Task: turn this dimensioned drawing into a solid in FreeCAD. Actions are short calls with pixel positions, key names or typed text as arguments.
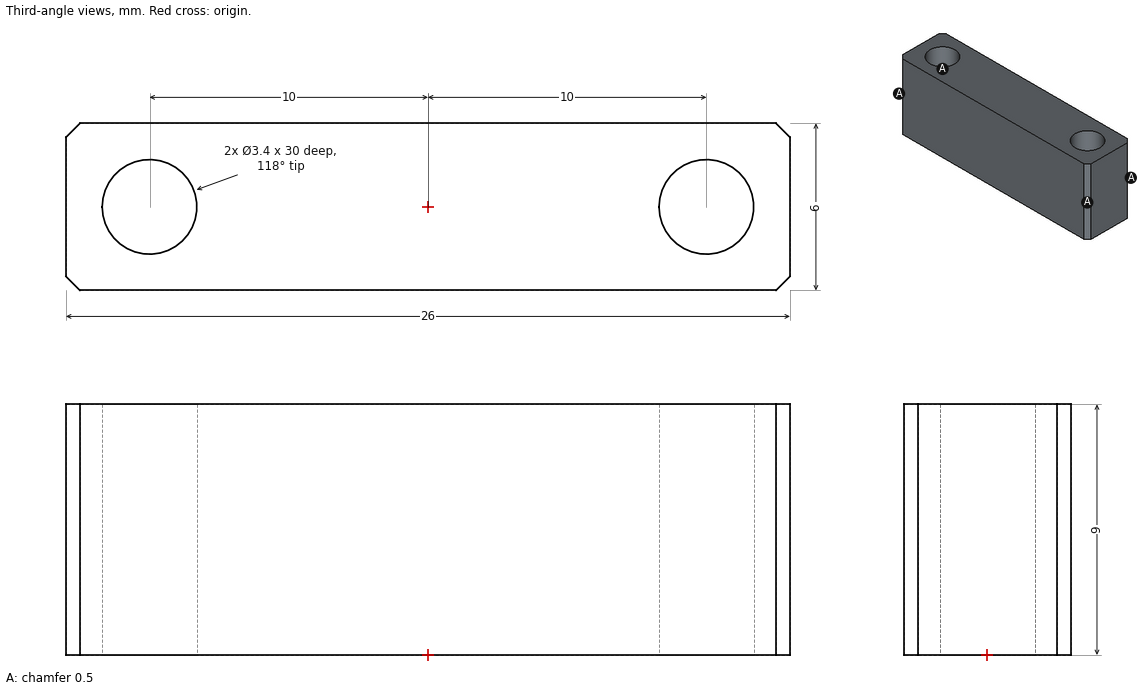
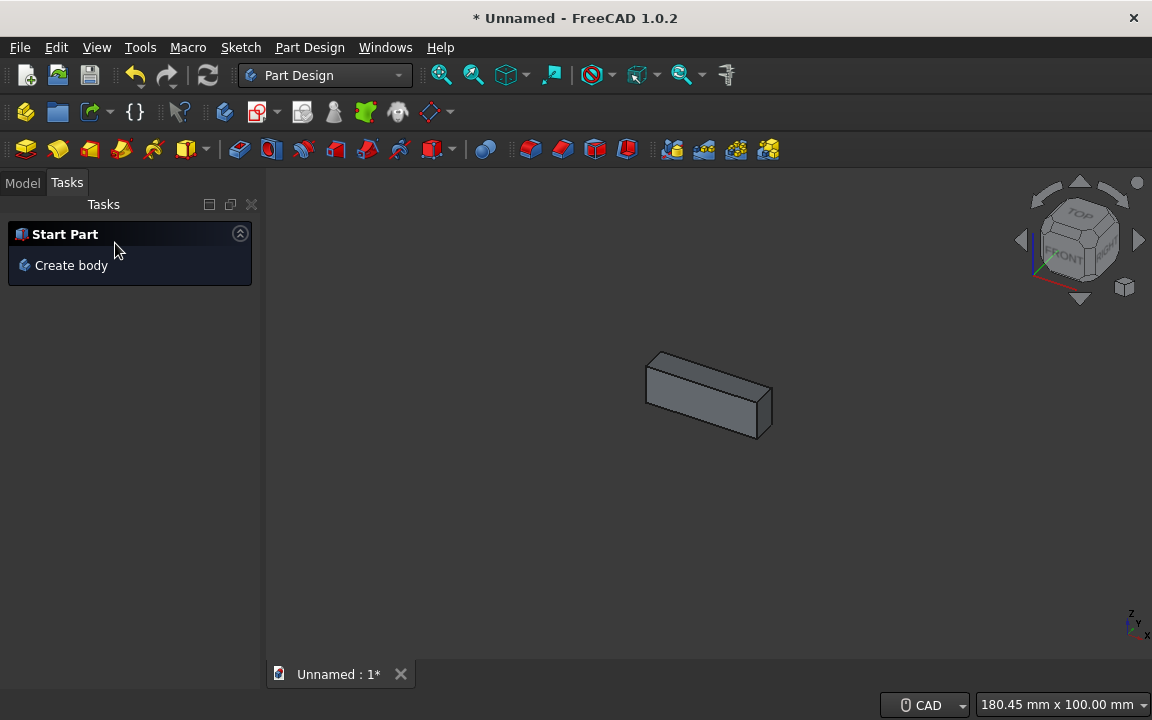
key(v)
key(f)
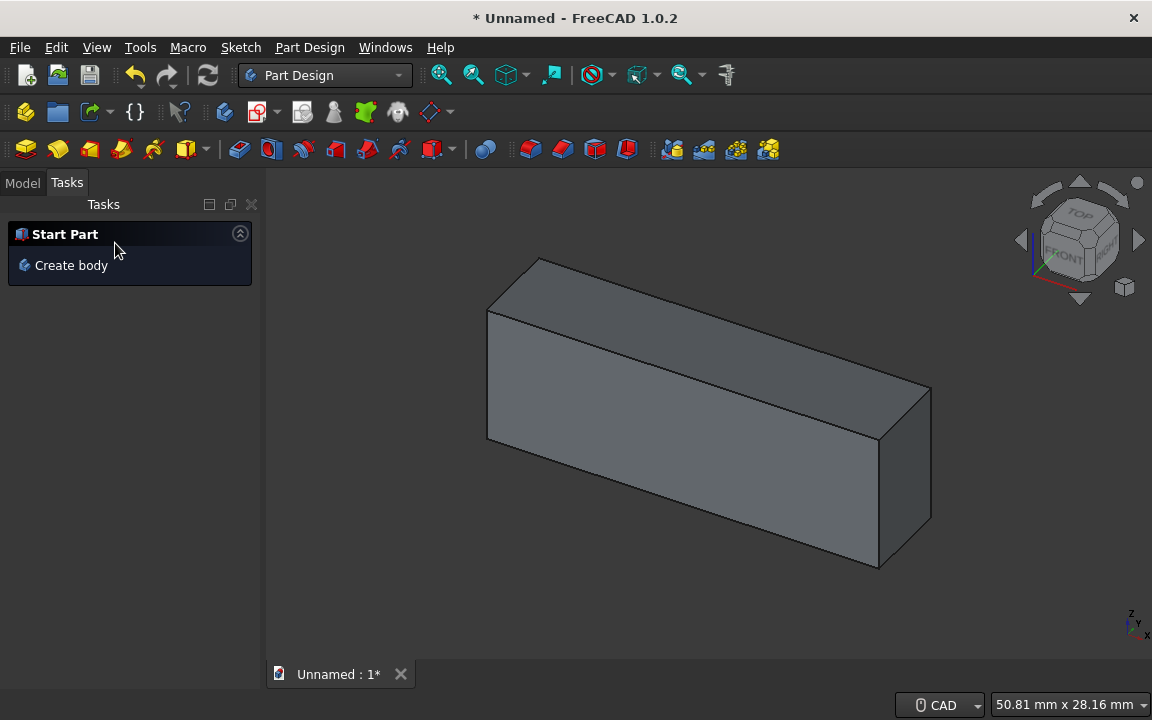
click(821, 385)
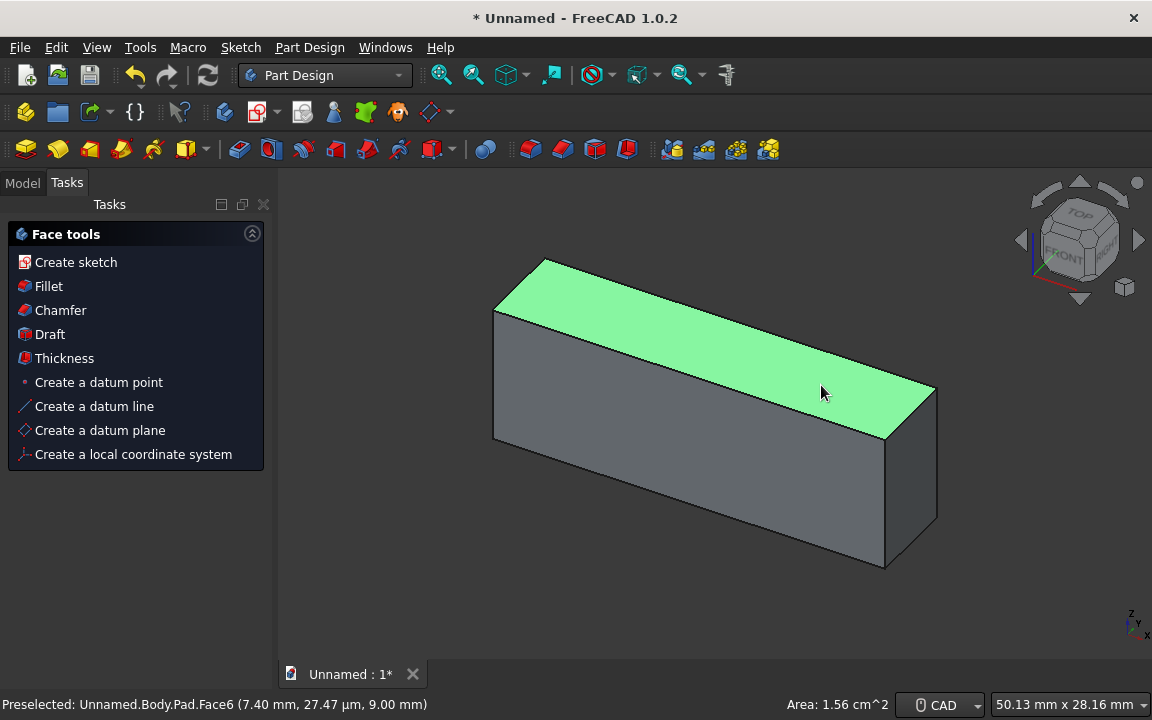
click(258, 112)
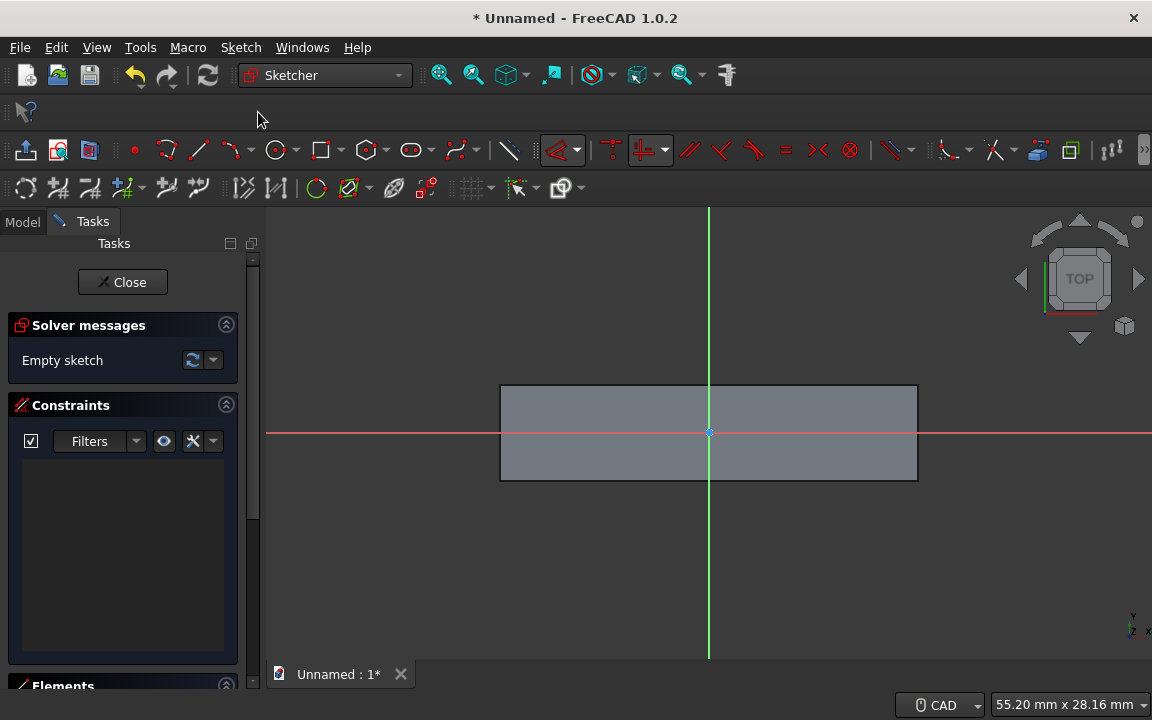
click(276, 150)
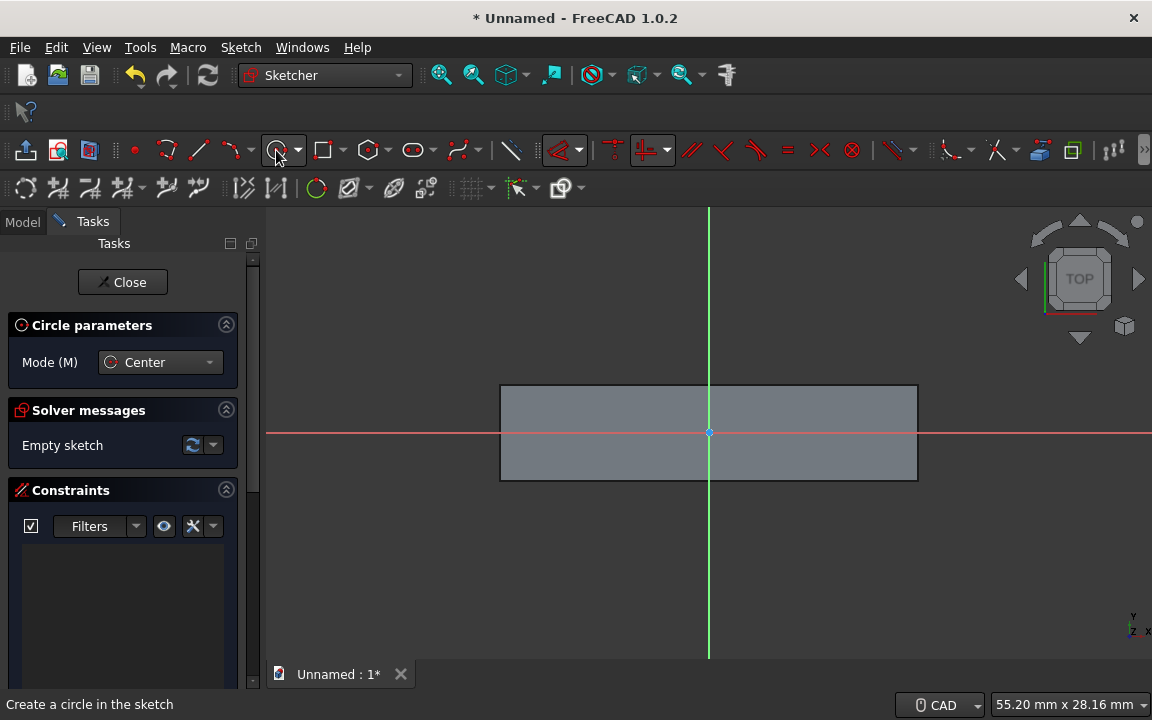
click(548, 433)
move(568, 414)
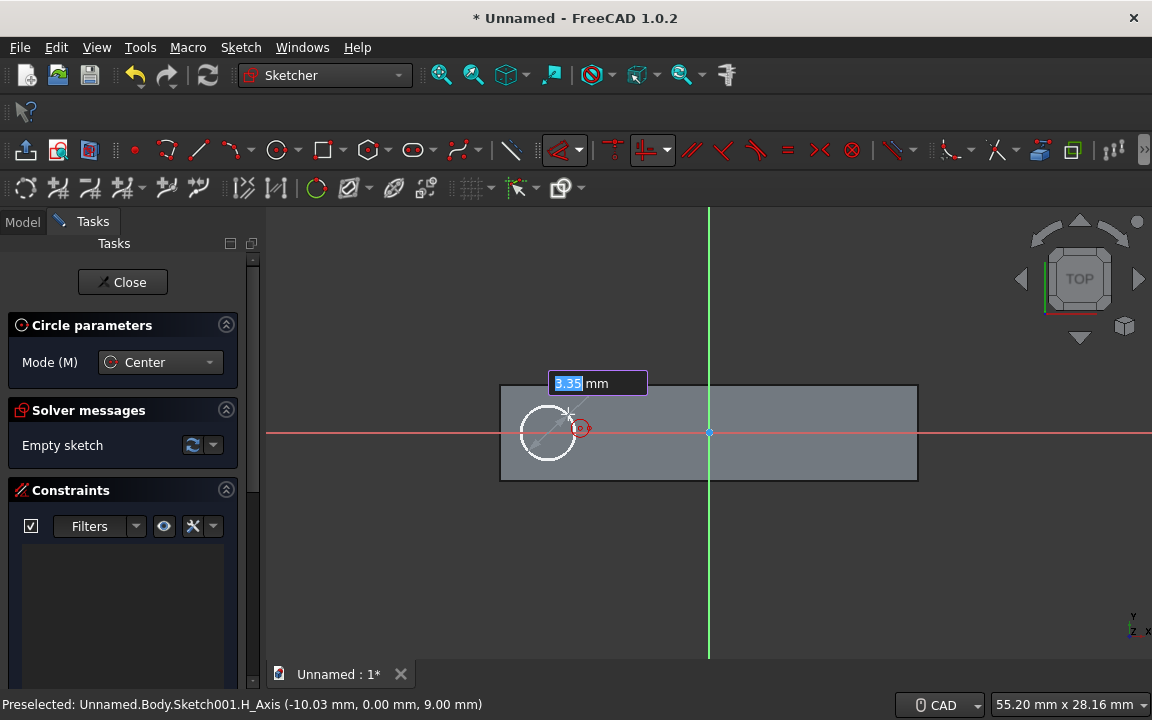
text(3.4)
key(Return)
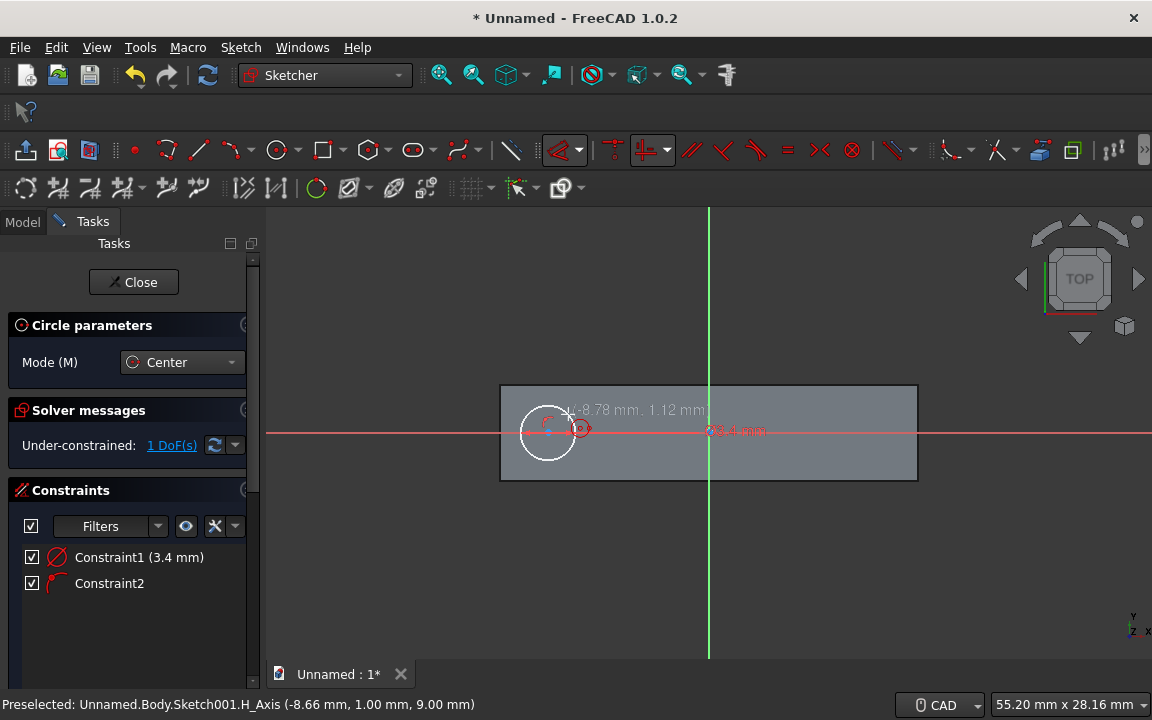
click(870, 433)
move(889, 414)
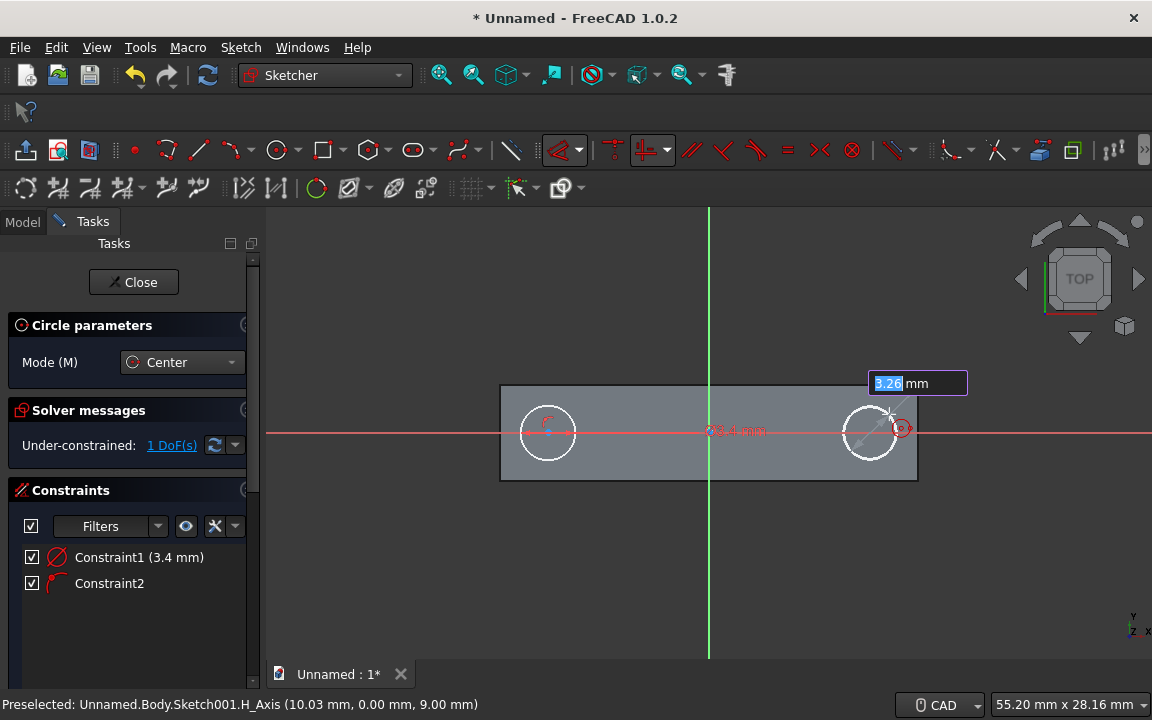
text(3.4)
key(Return)
key(Escape)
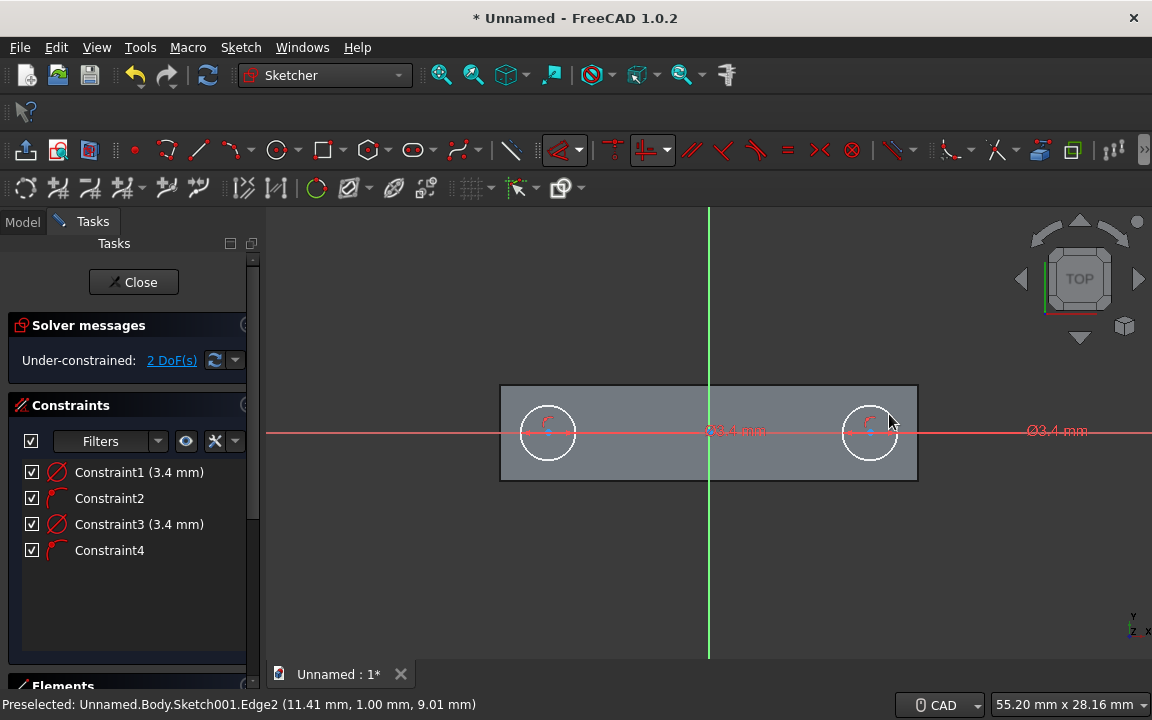
key(d)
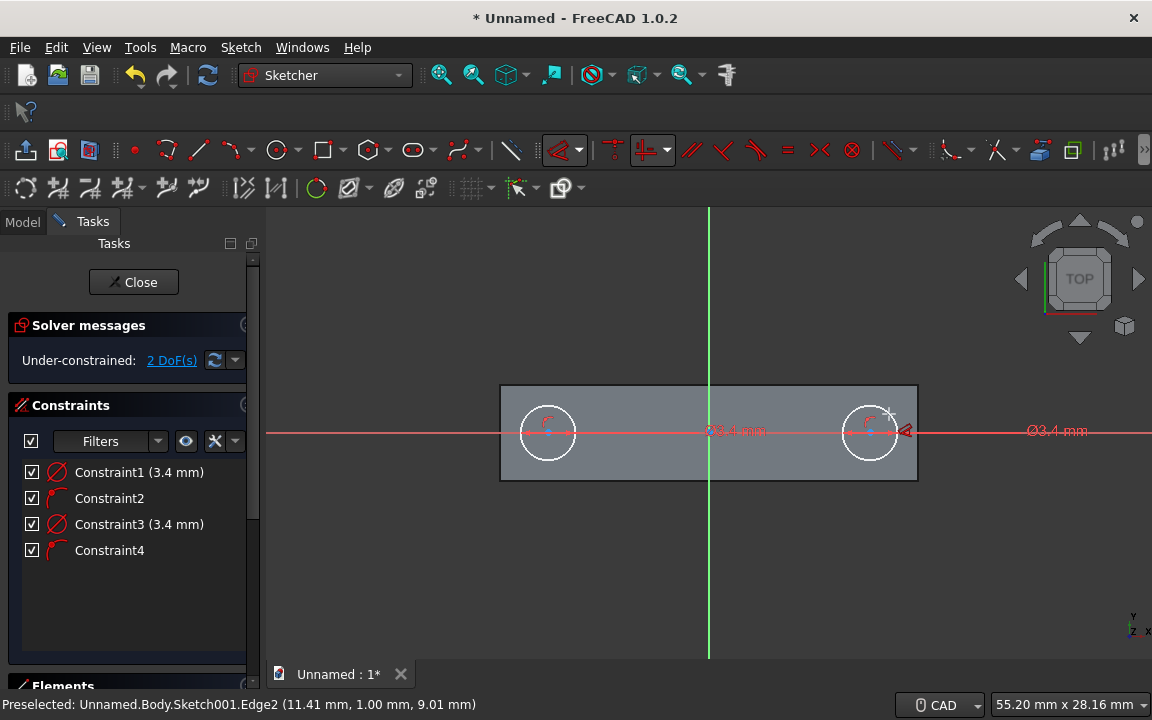
click(548, 433)
click(629, 467)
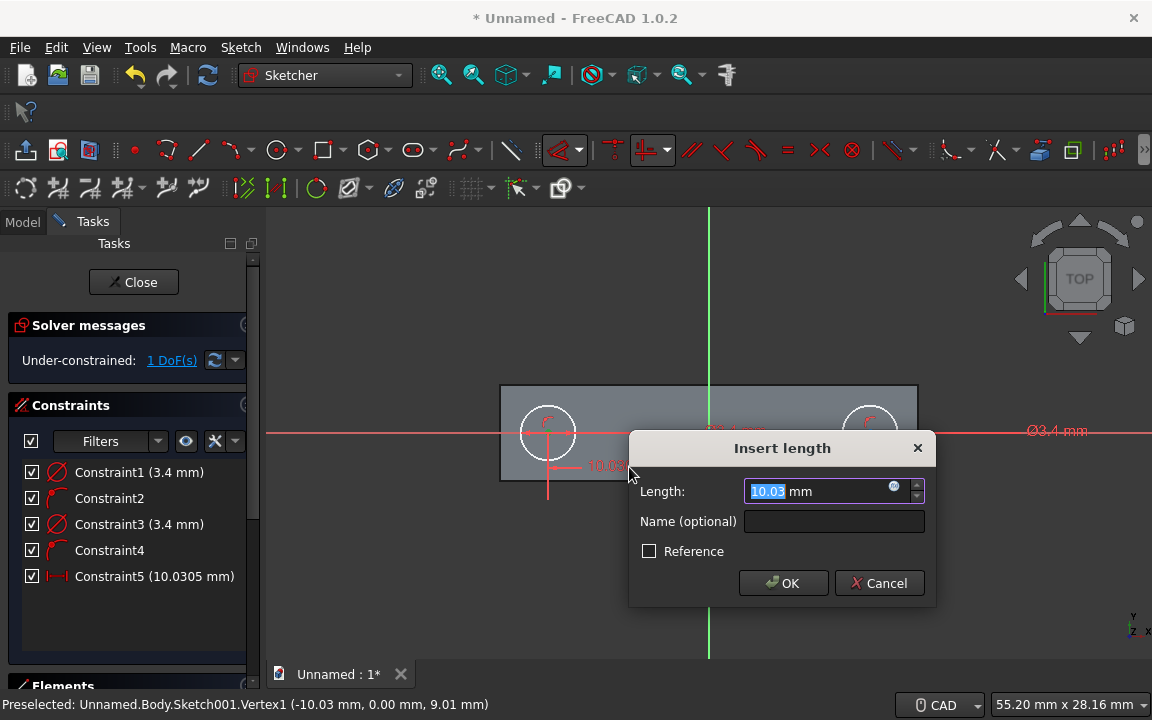
text(10)
key(Return)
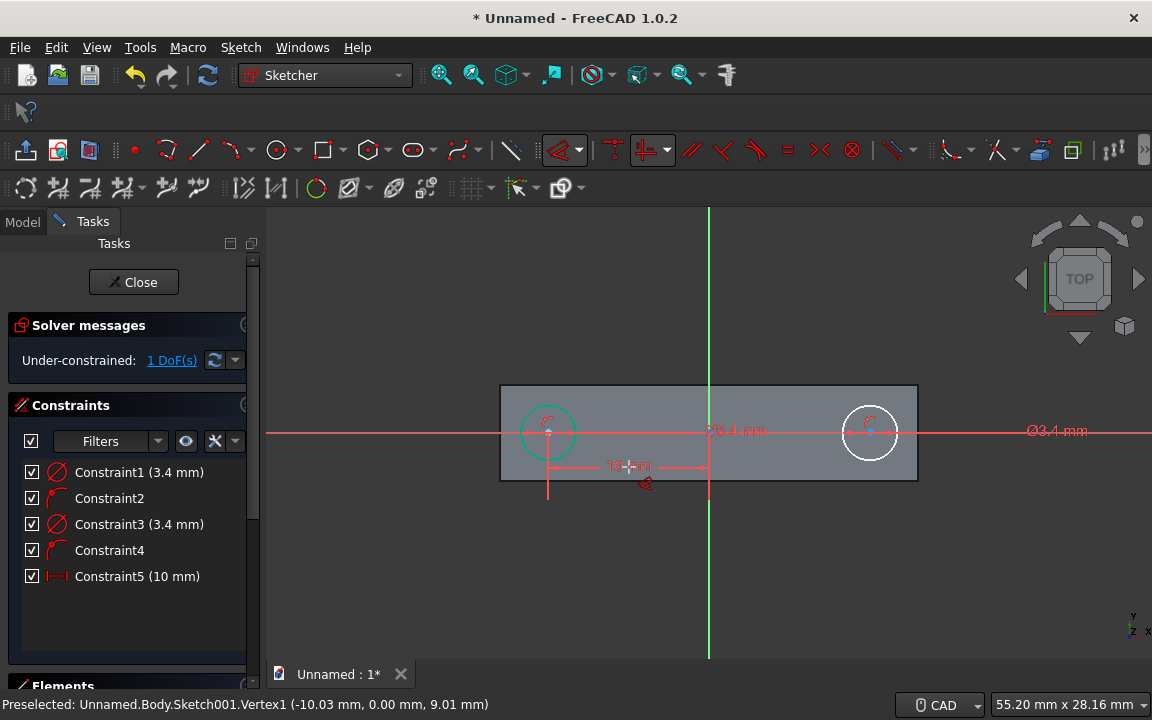
click(870, 433)
click(789, 467)